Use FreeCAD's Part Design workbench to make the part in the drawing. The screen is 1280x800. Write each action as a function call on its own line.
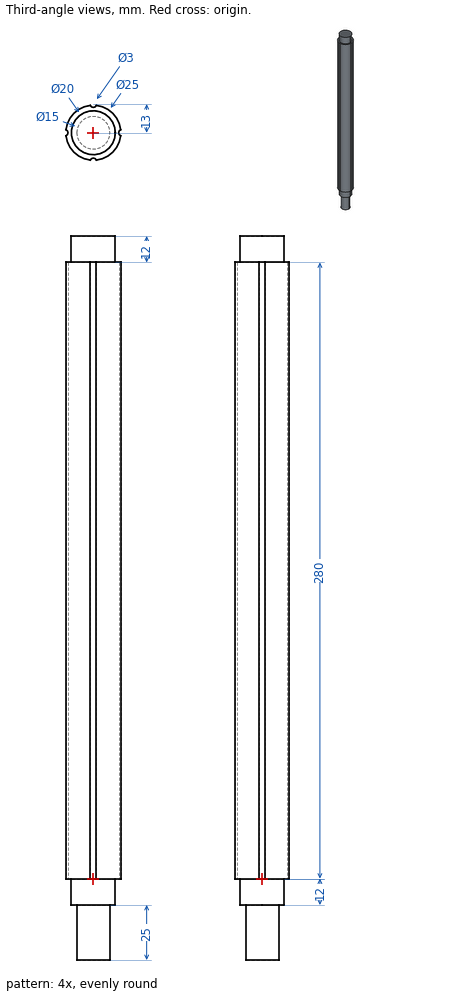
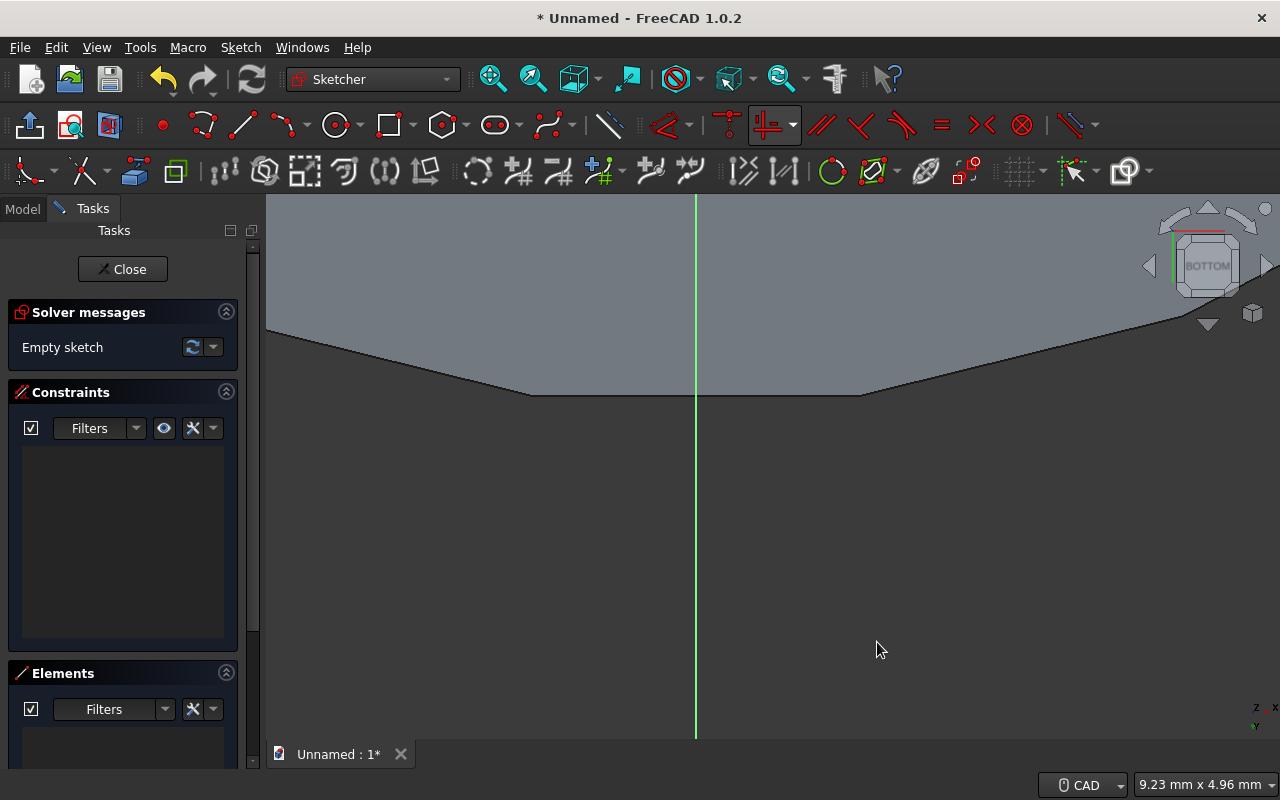
key(g)
key(c)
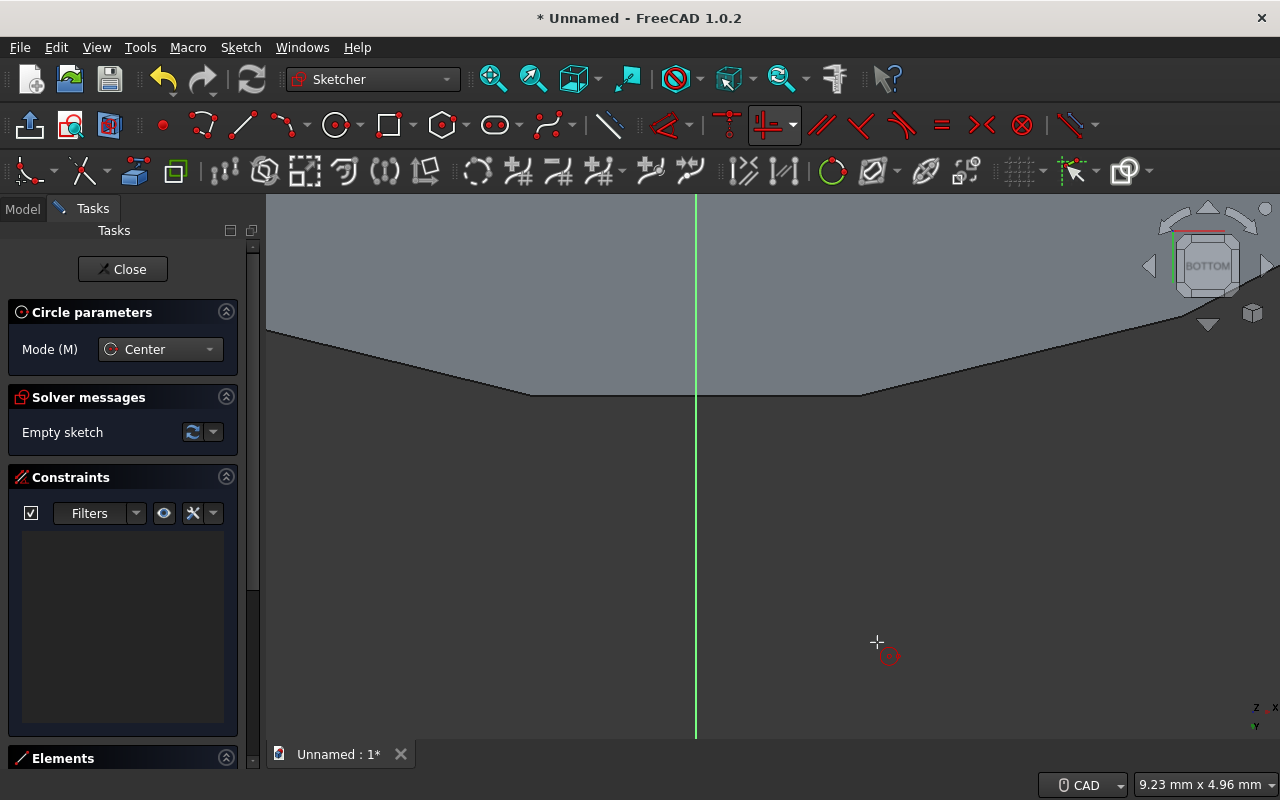
click(696, 460)
click(813, 344)
key(Escape)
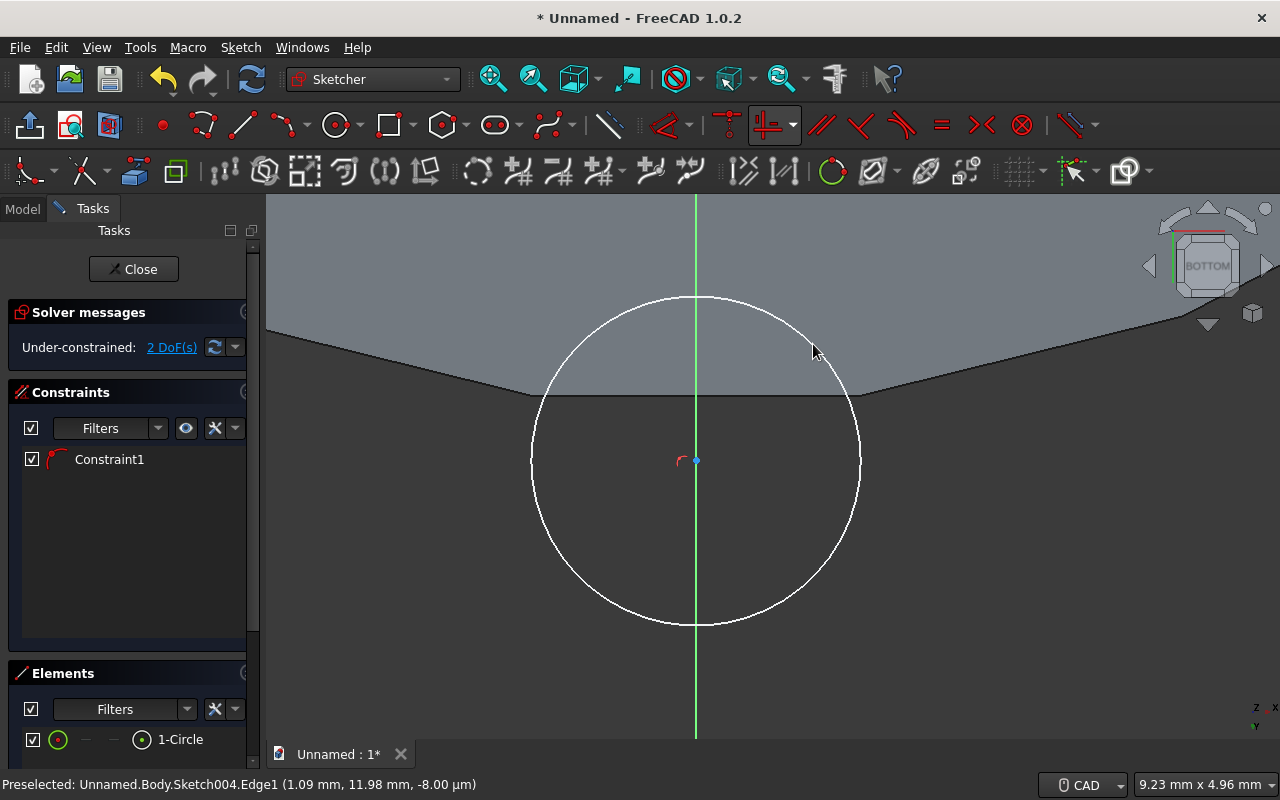
click(664, 126)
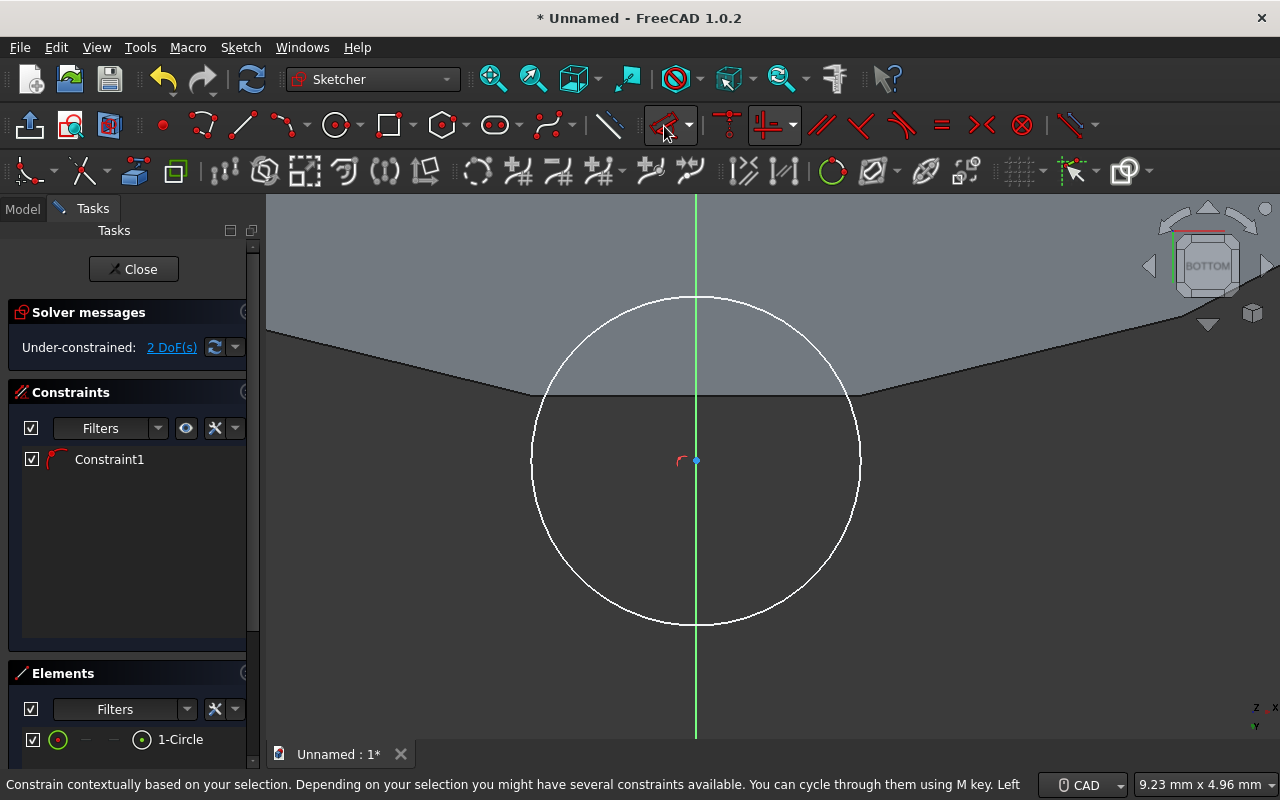
click(812, 344)
click(835, 321)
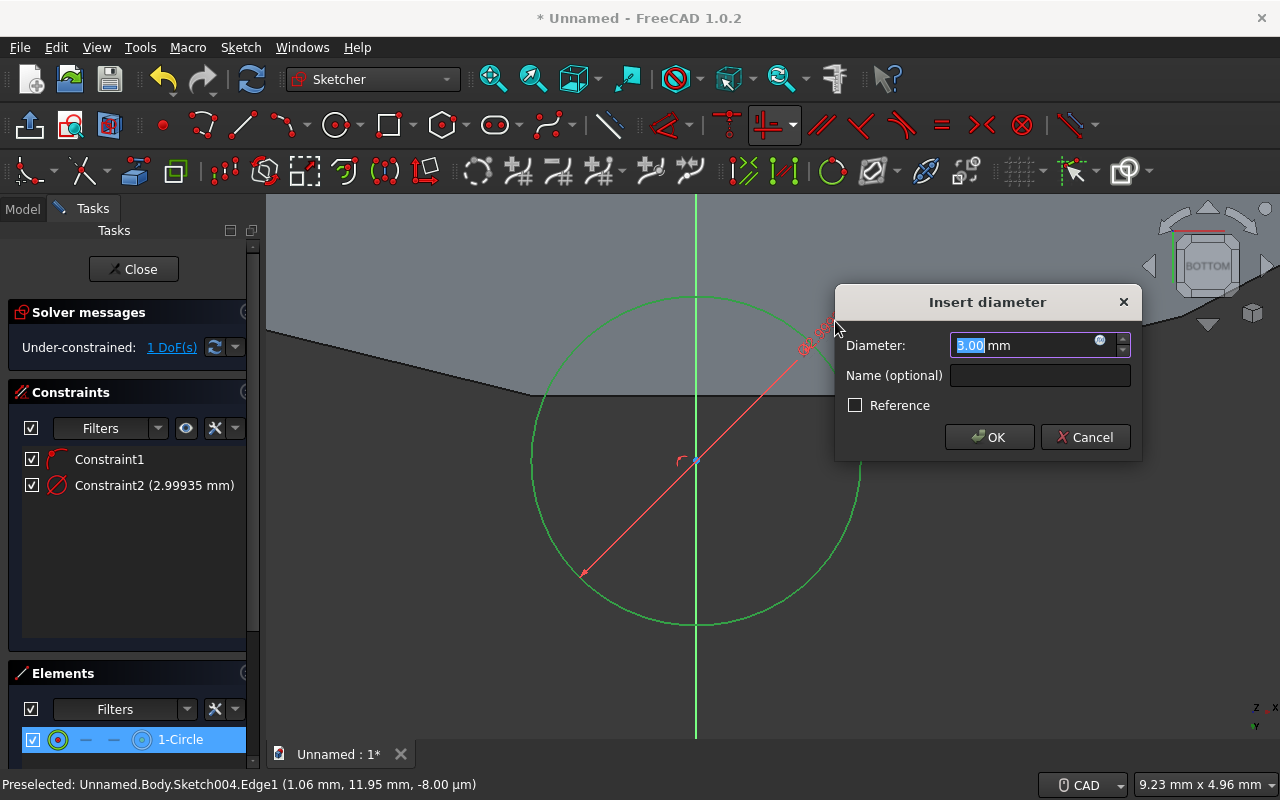
text(3)
key(Return)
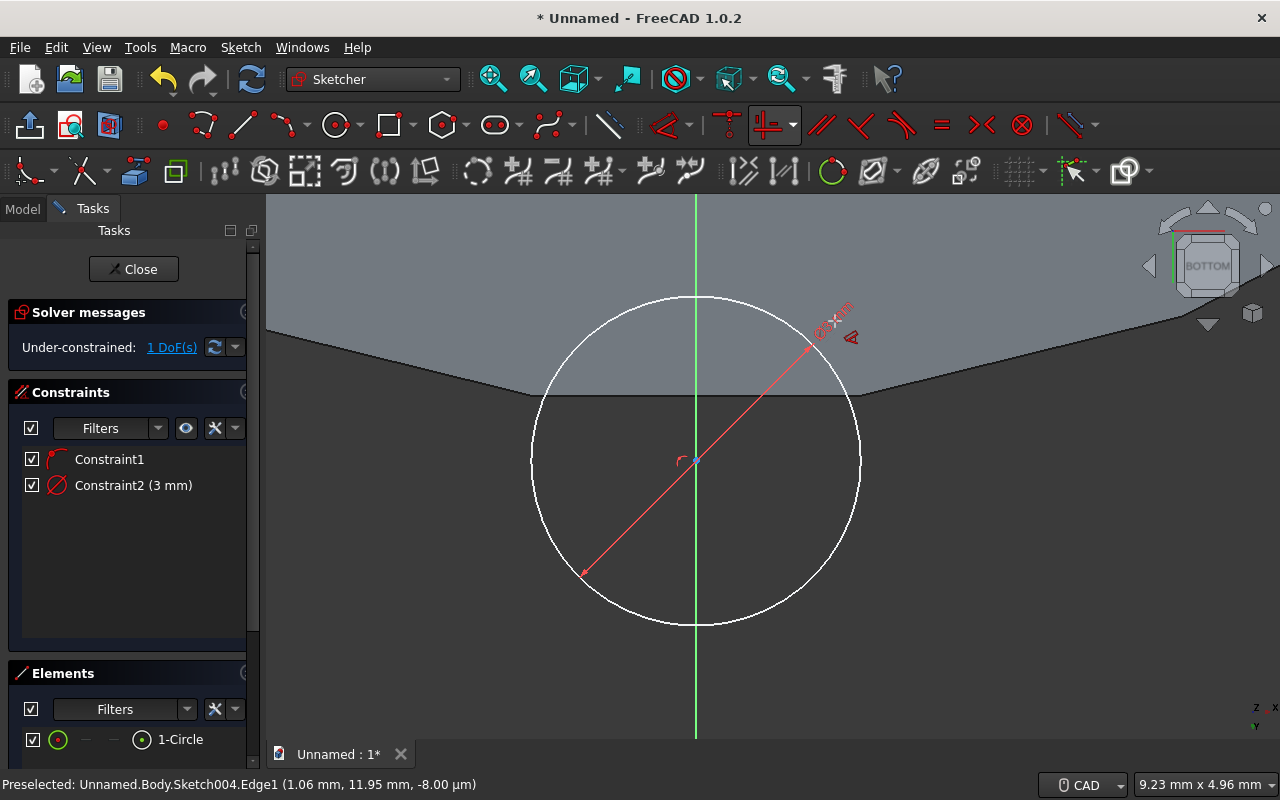
click(696, 461)
click(730, 341)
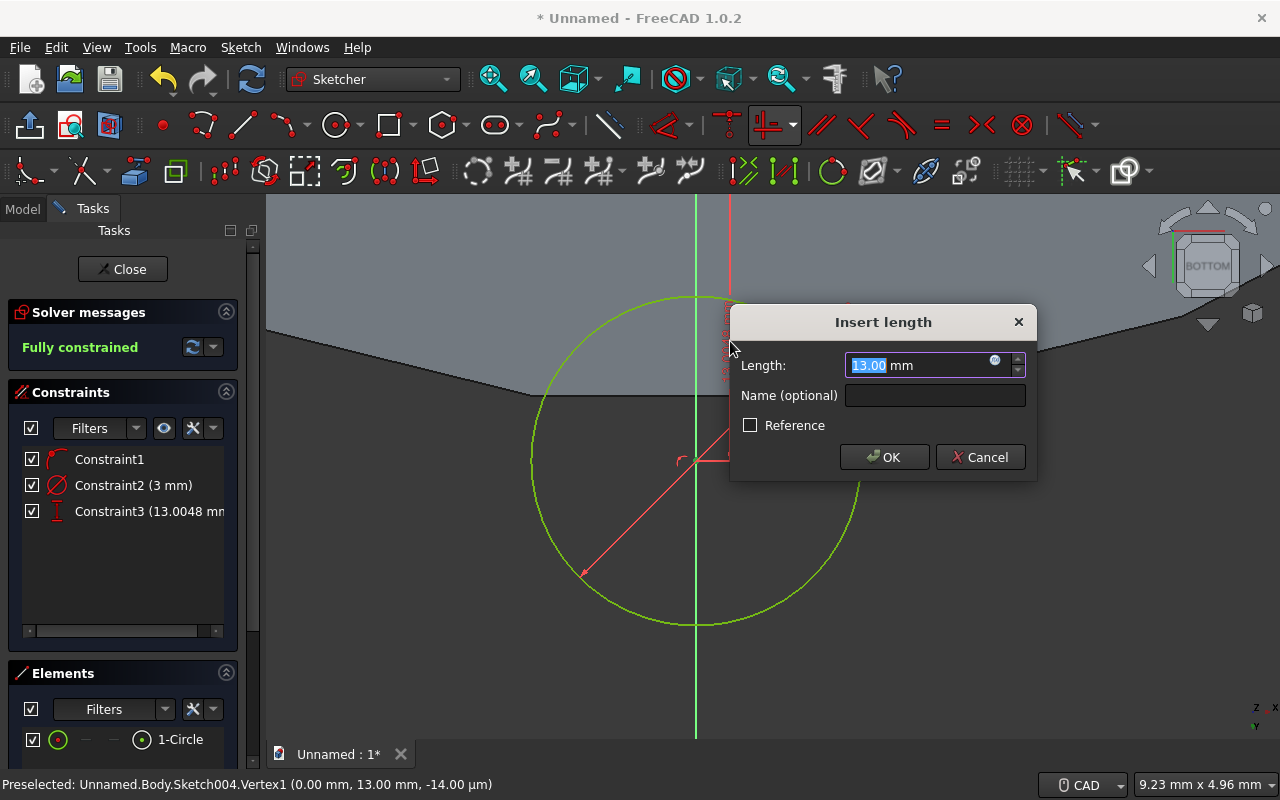
text(13)
key(Return)
key(Escape)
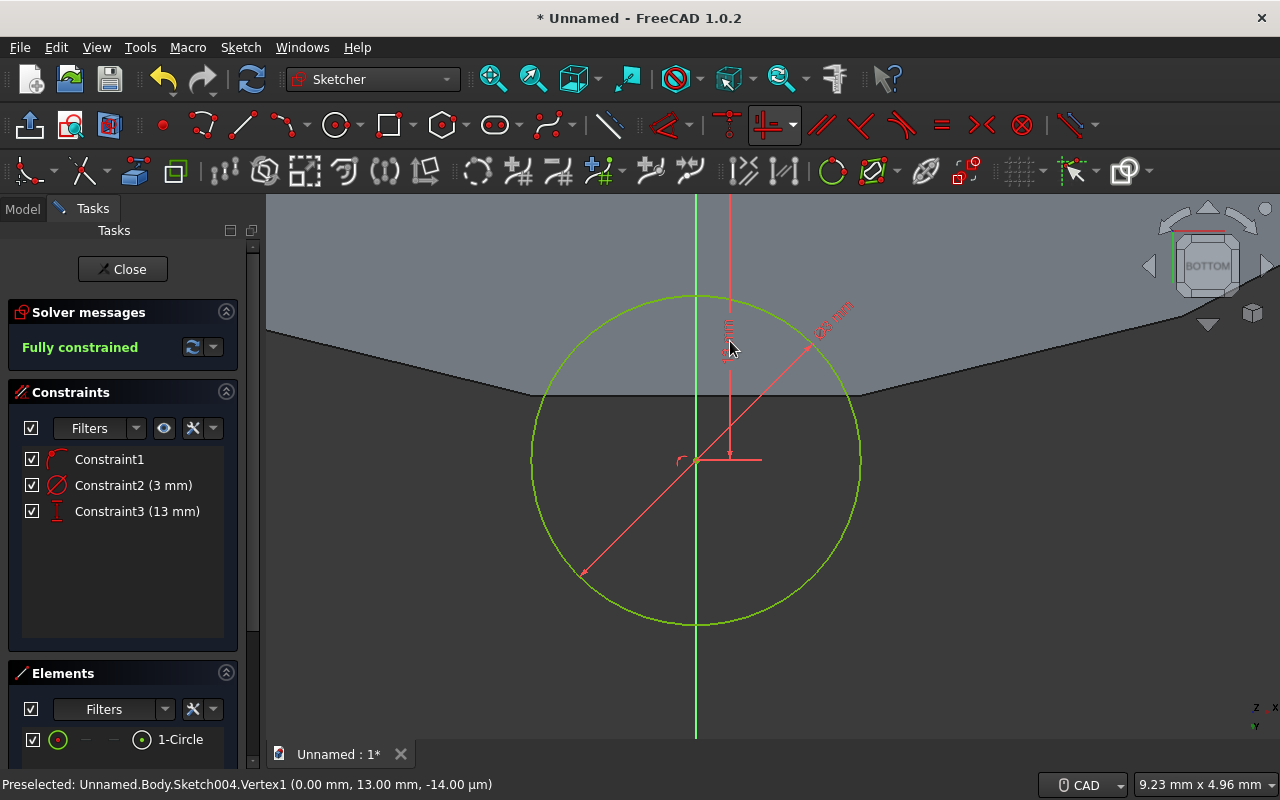
click(123, 269)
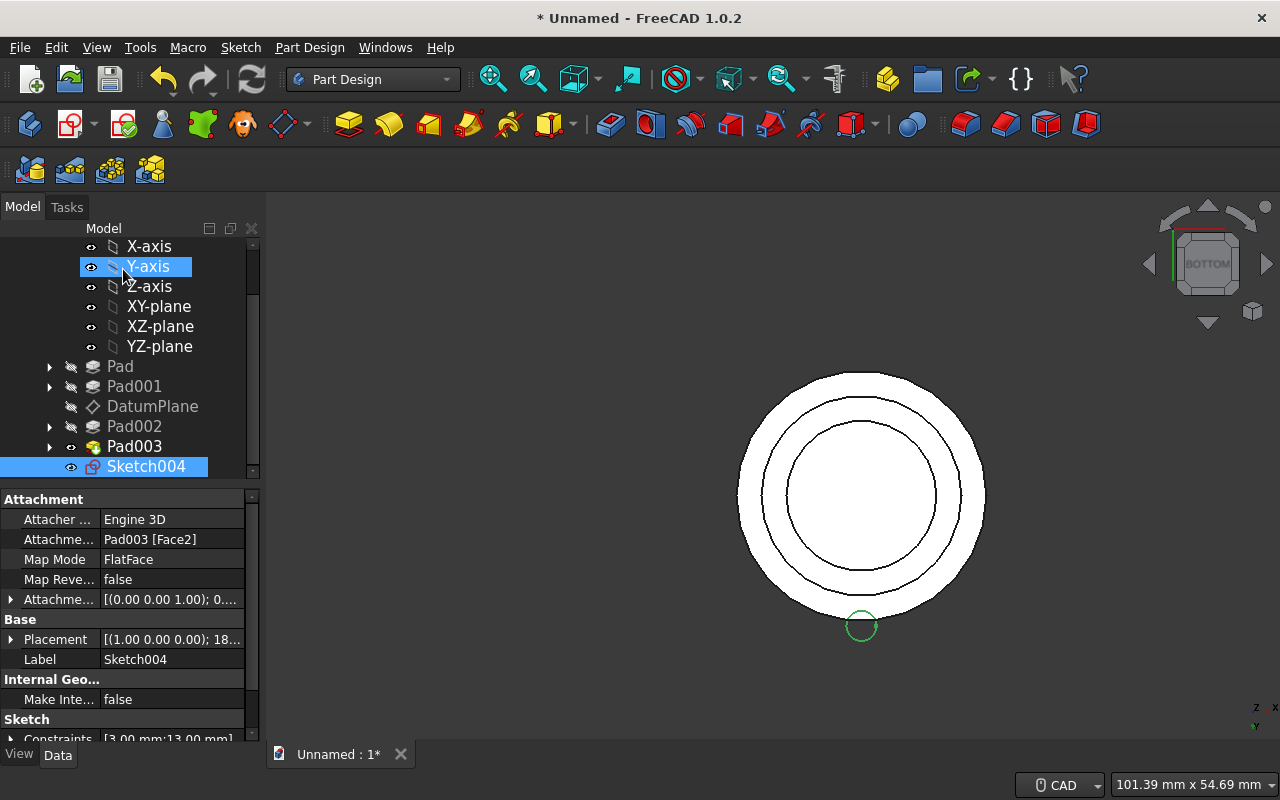
click(612, 124)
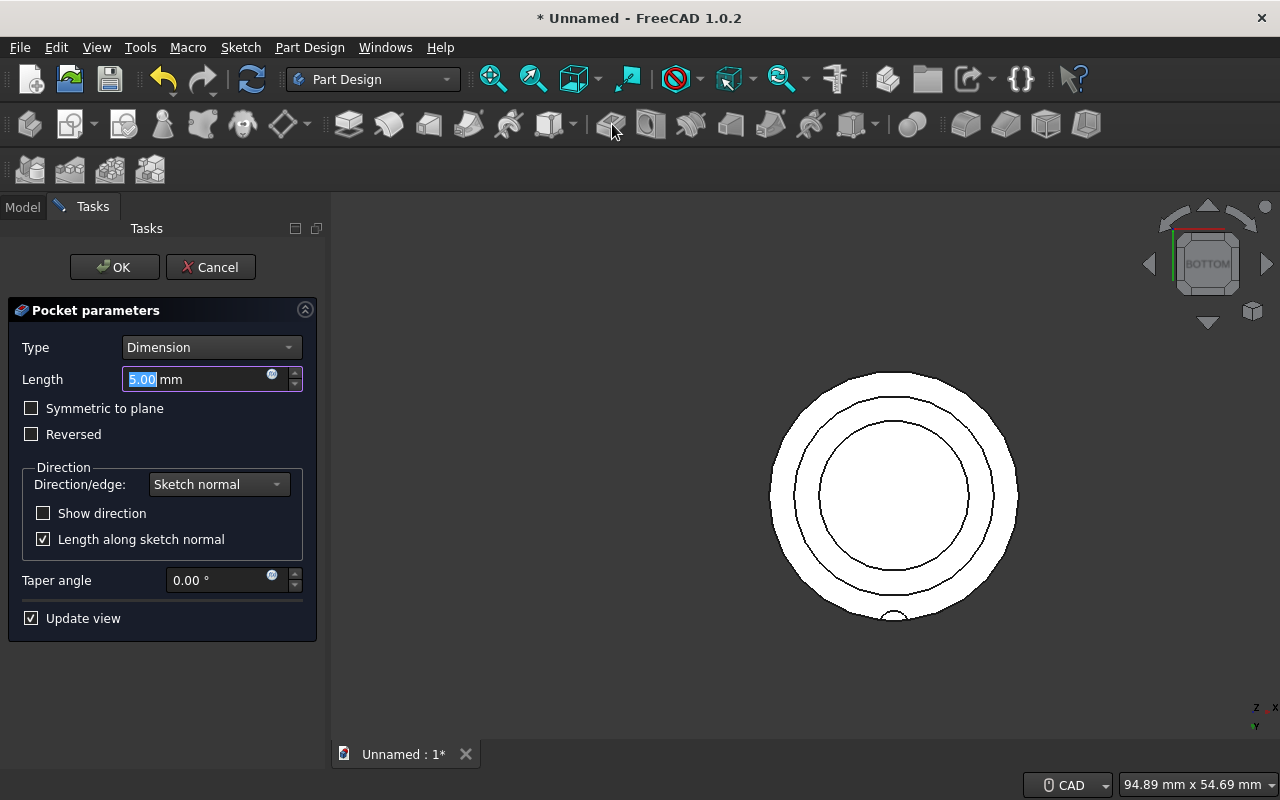
text(280)
key(Tab)